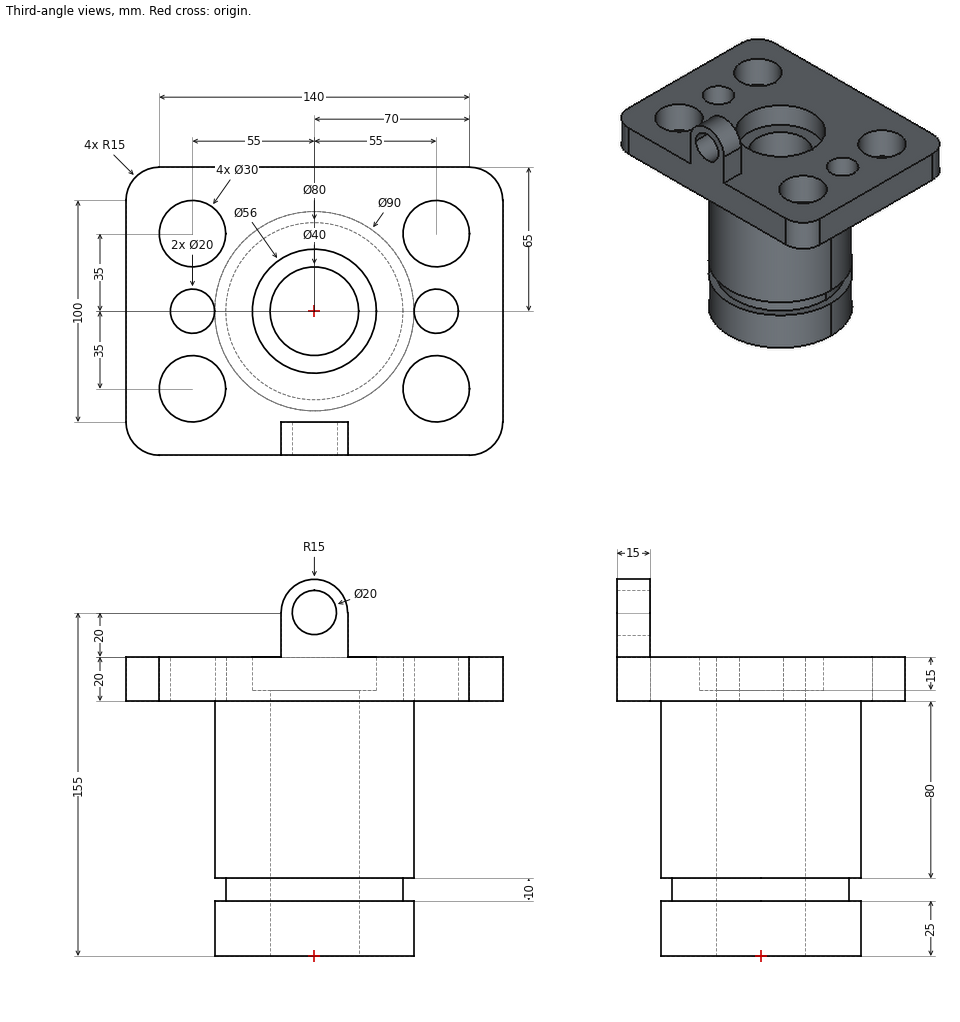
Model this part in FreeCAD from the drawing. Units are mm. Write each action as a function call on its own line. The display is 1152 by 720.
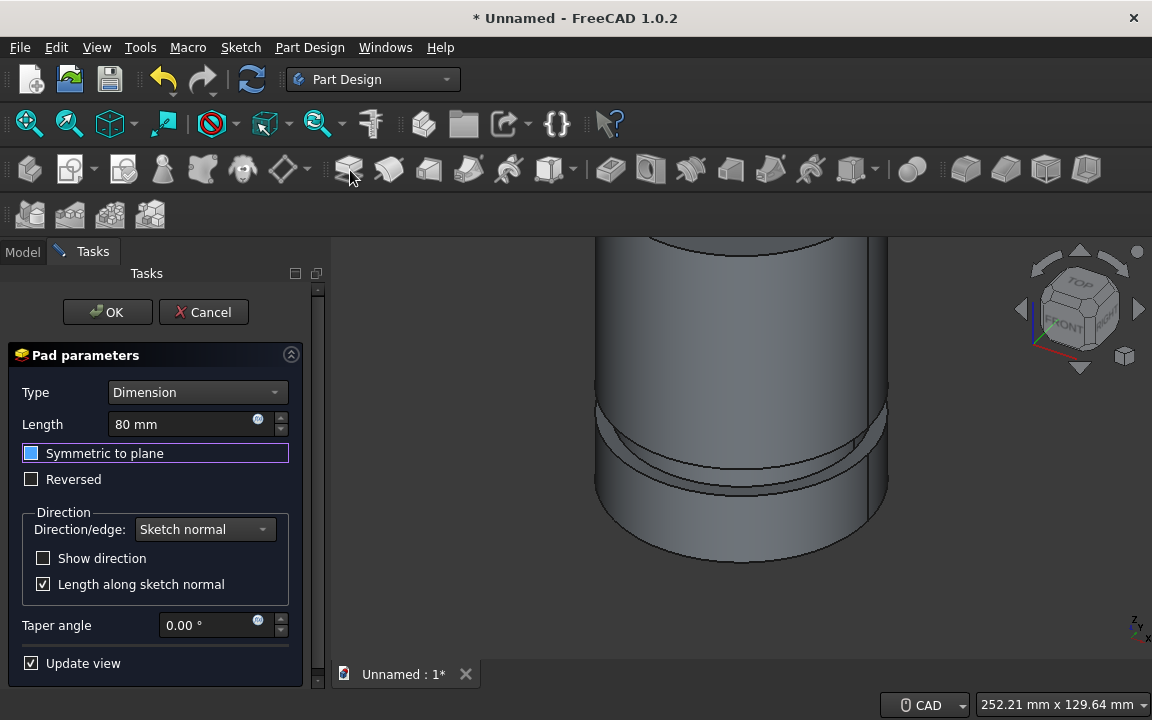
click(108, 312)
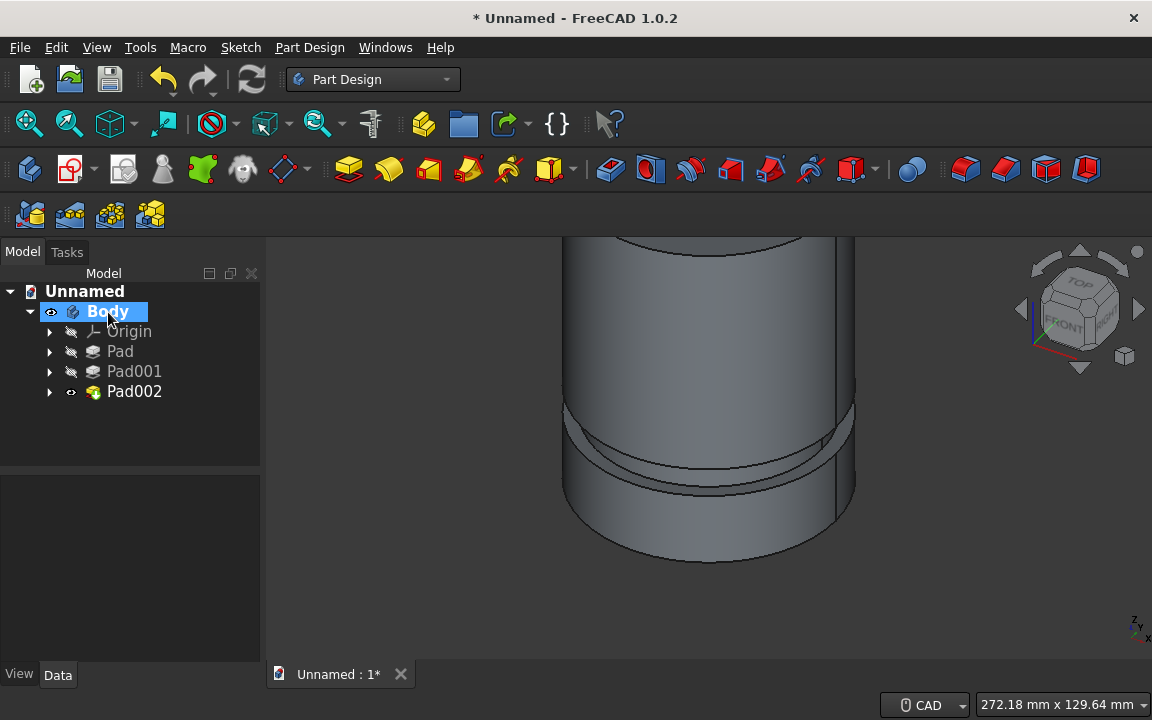
click(30, 124)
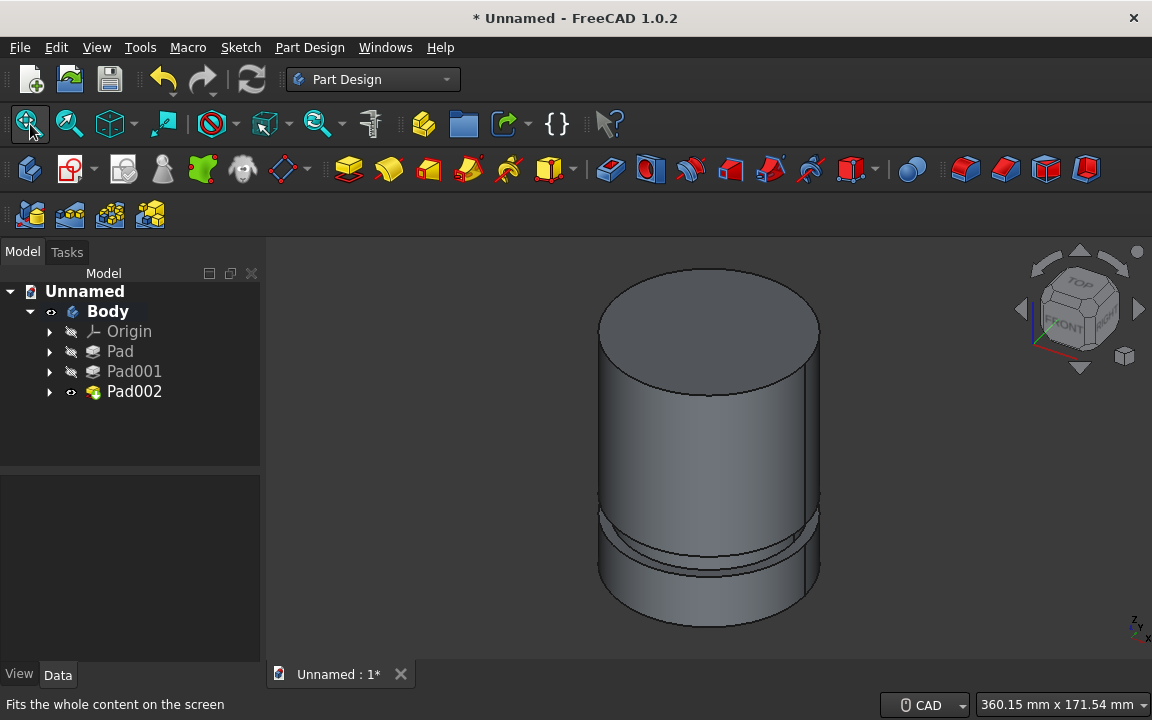
click(709, 331)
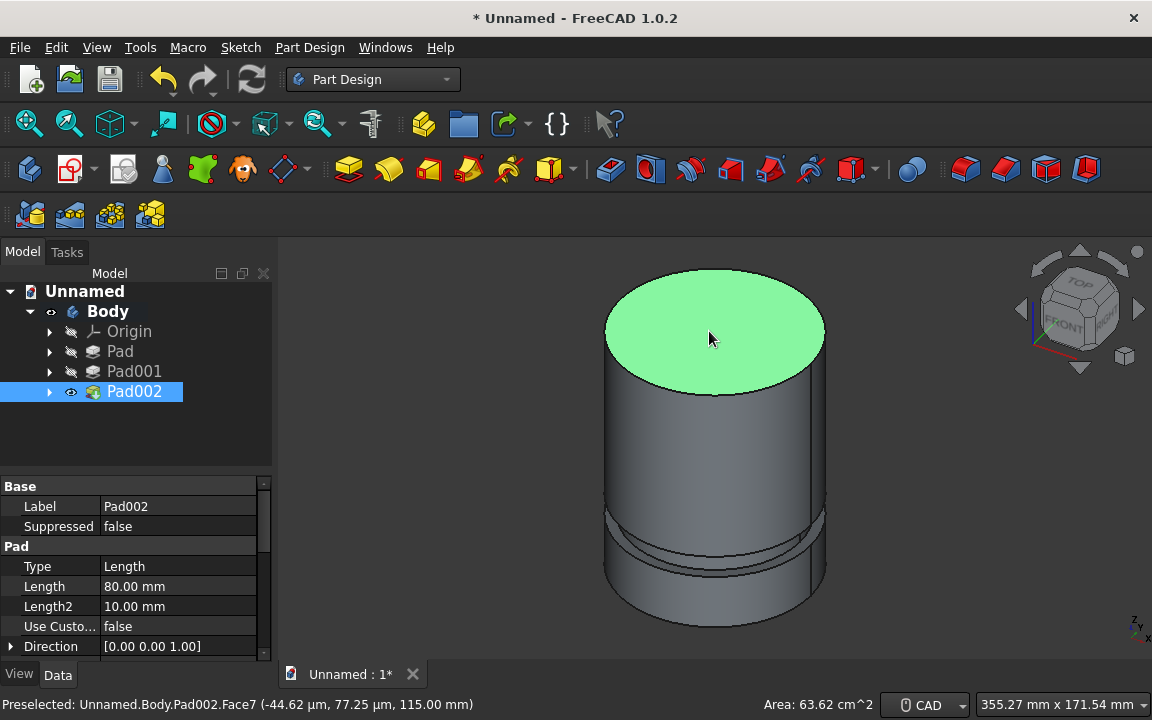
click(70, 170)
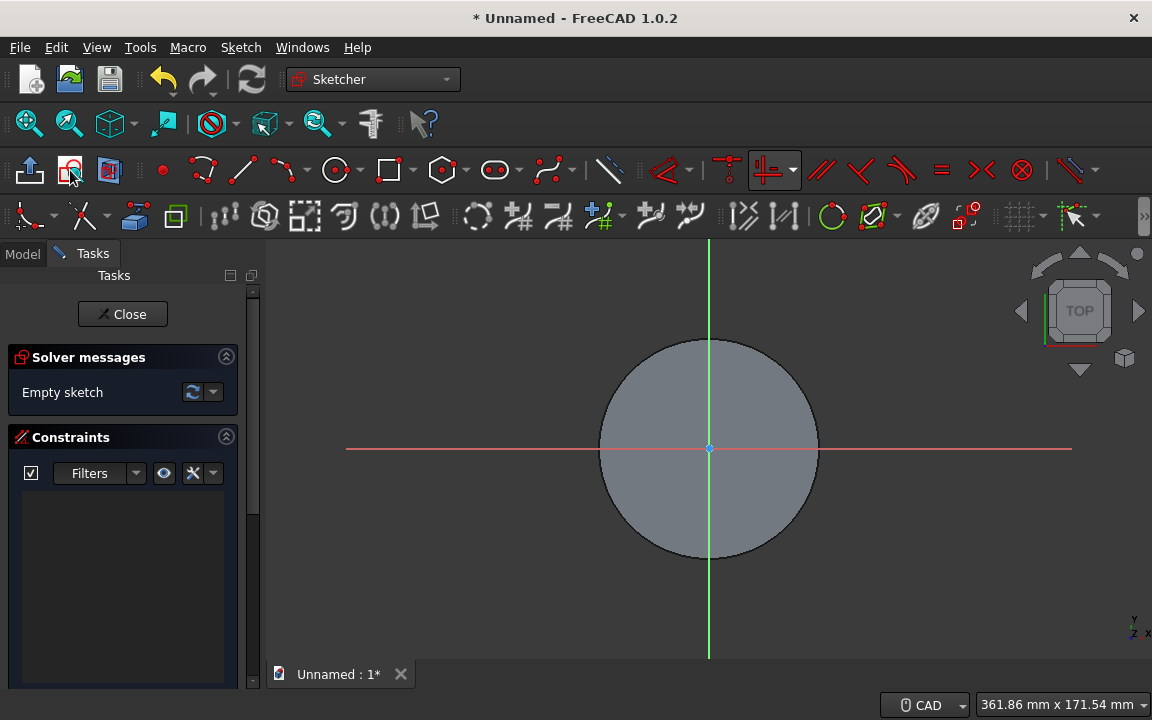
scroll(331, 449, down, 1)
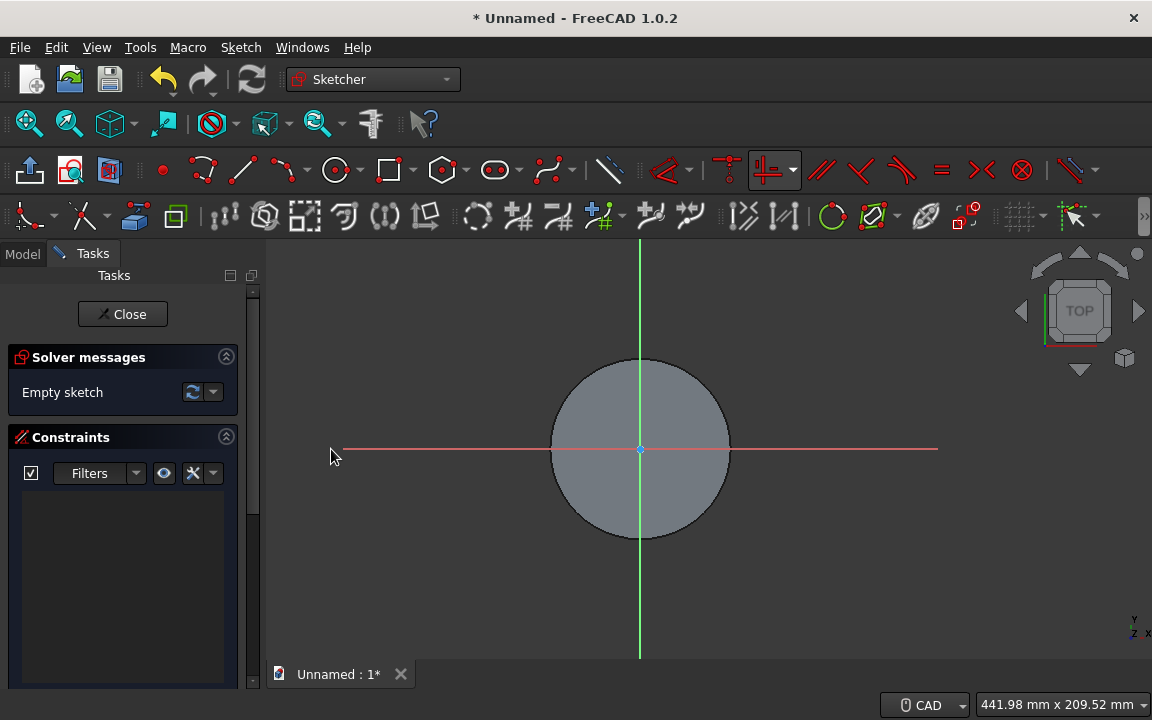
click(244, 170)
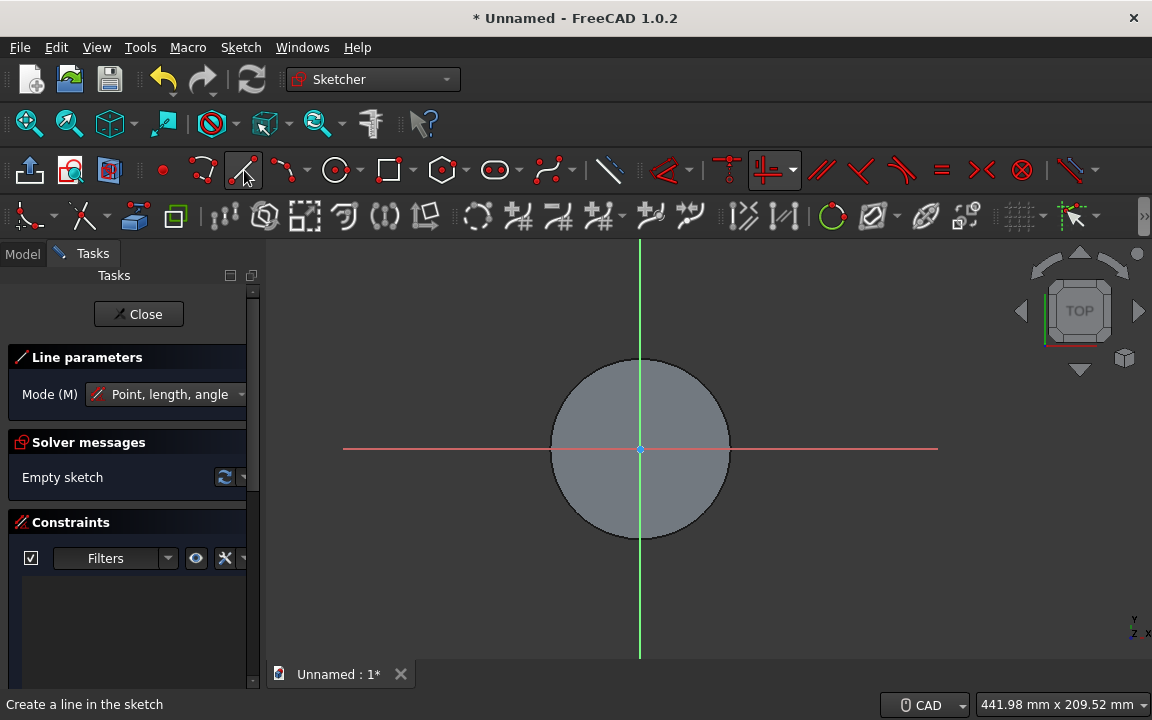
click(781, 319)
click(500, 319)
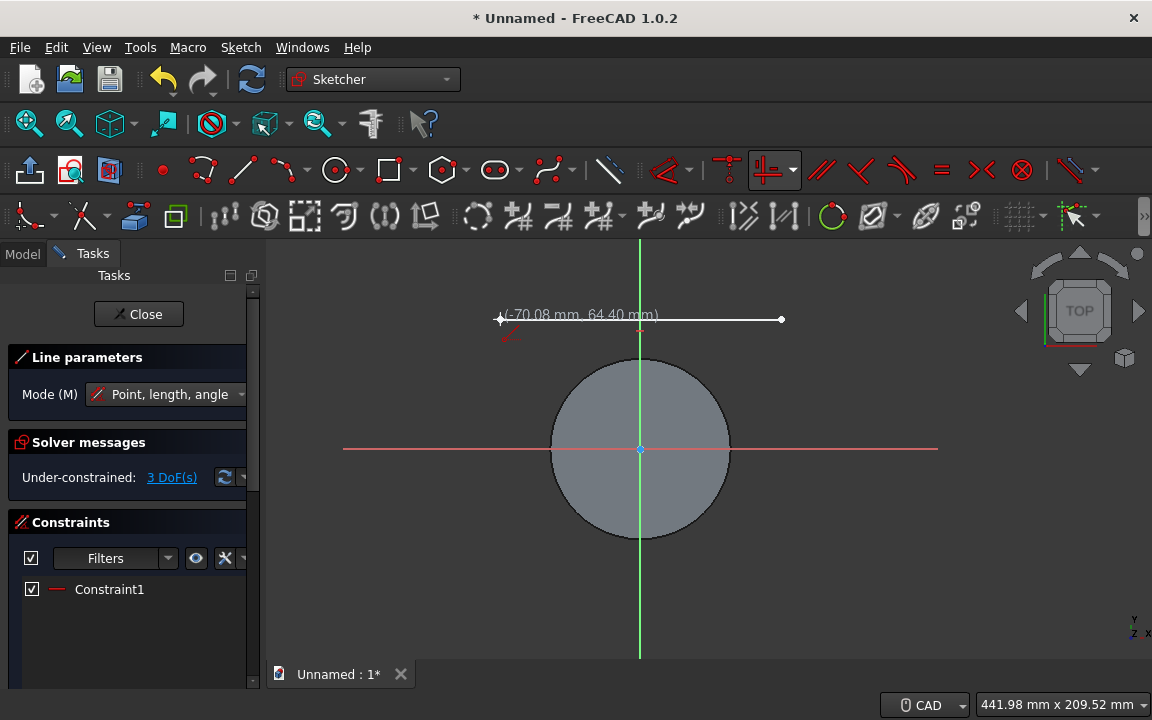
click(470, 349)
click(470, 549)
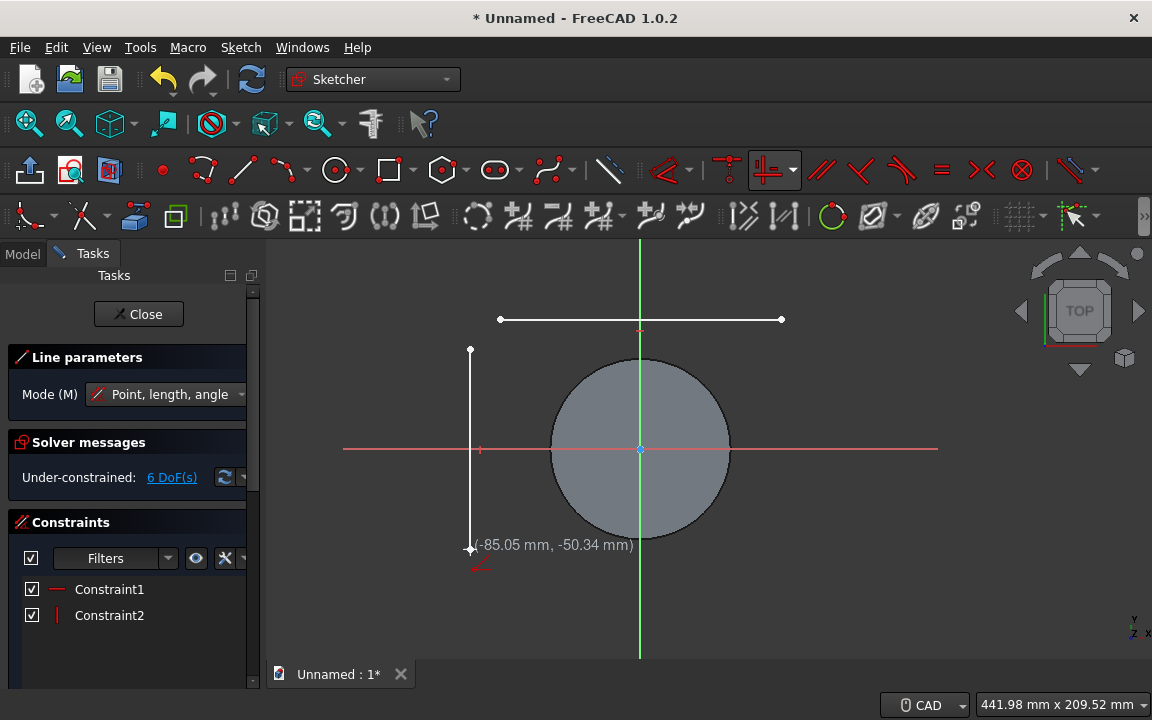
click(500, 579)
click(781, 579)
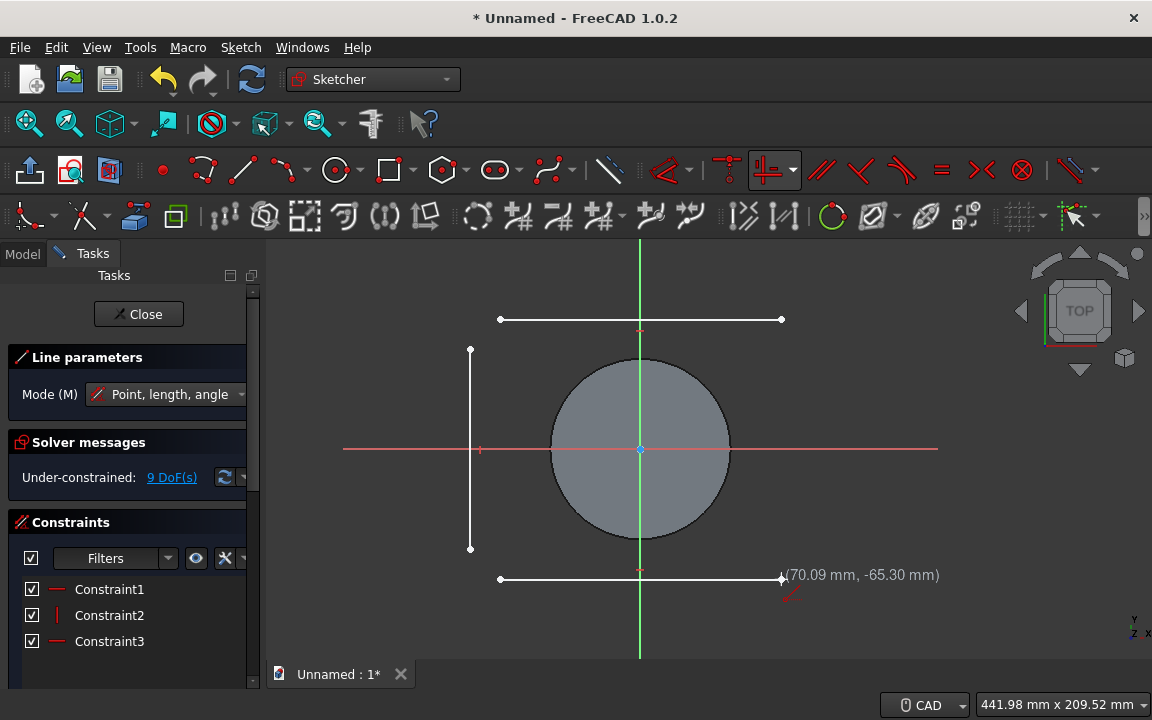
click(811, 549)
click(811, 349)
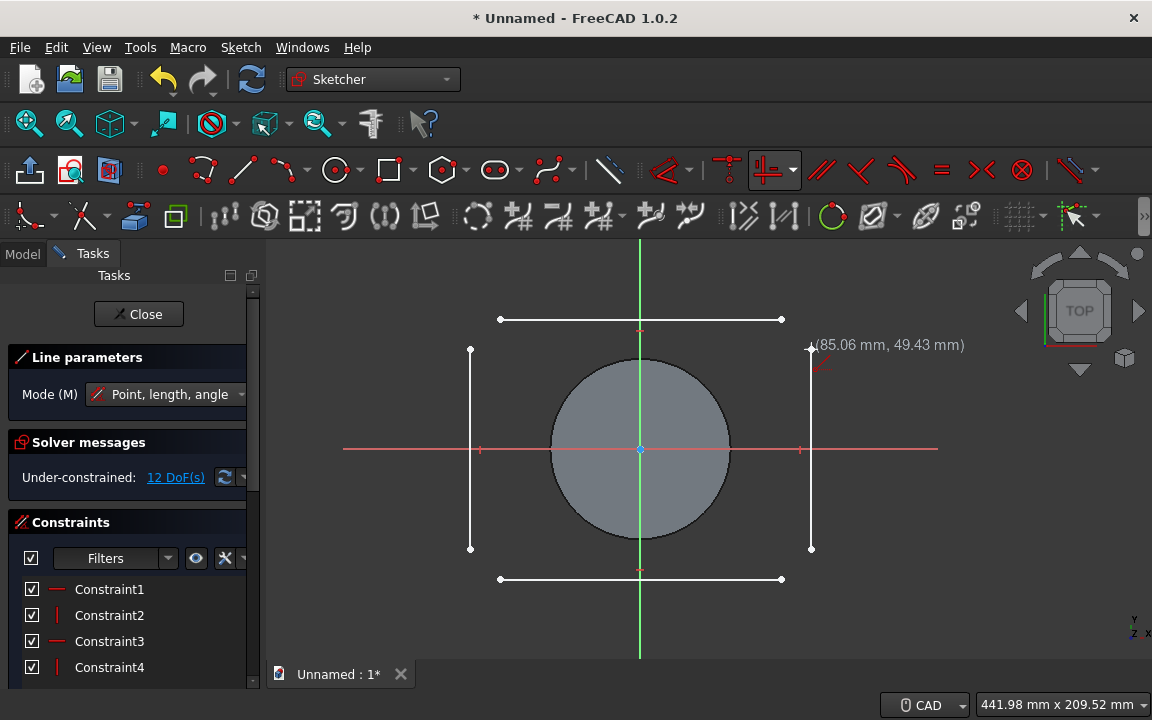
click(284, 170)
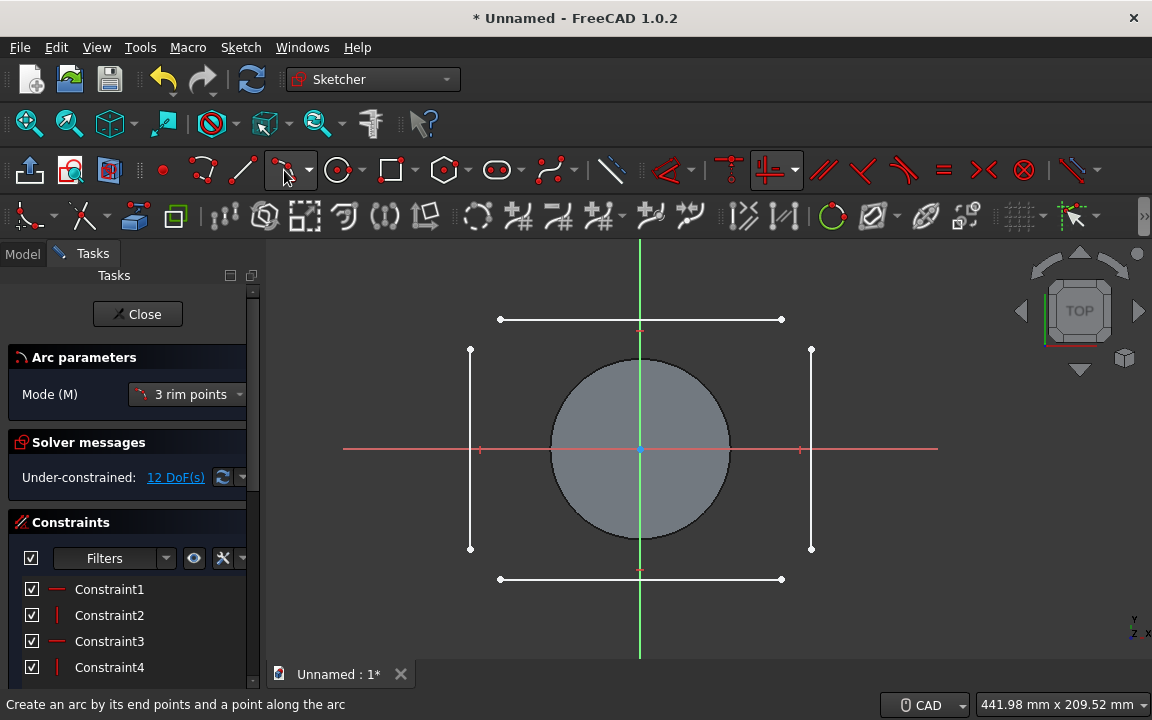
click(500, 320)
click(470, 350)